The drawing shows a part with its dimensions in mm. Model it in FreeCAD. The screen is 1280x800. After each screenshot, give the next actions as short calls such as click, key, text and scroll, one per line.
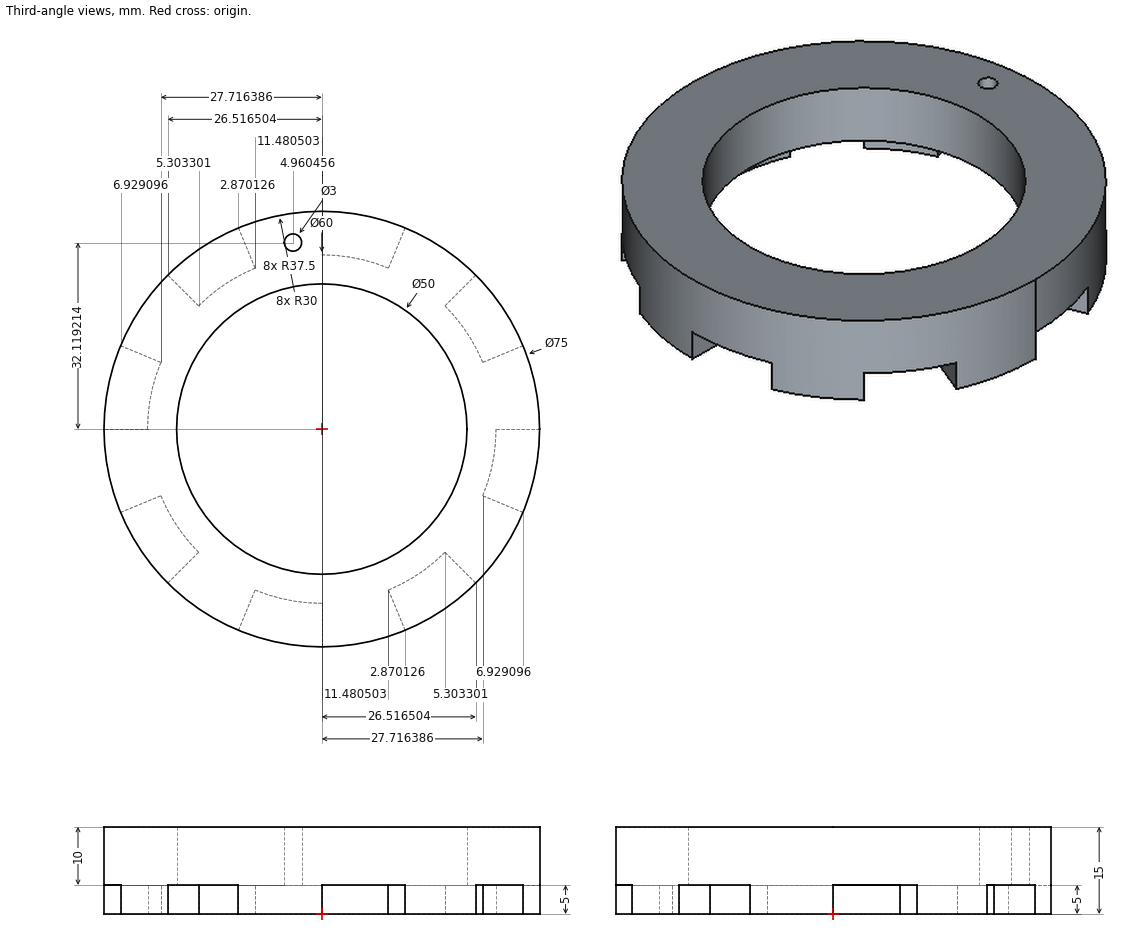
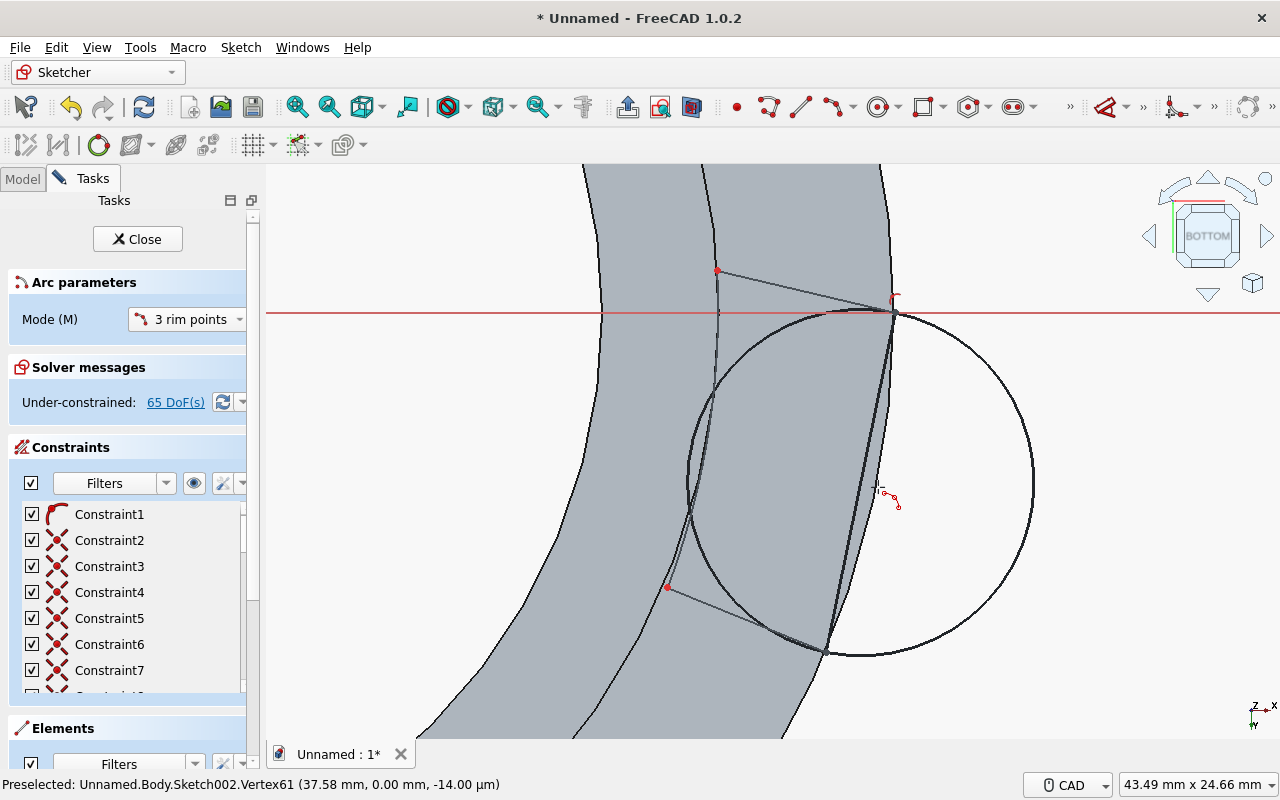
click(877, 484)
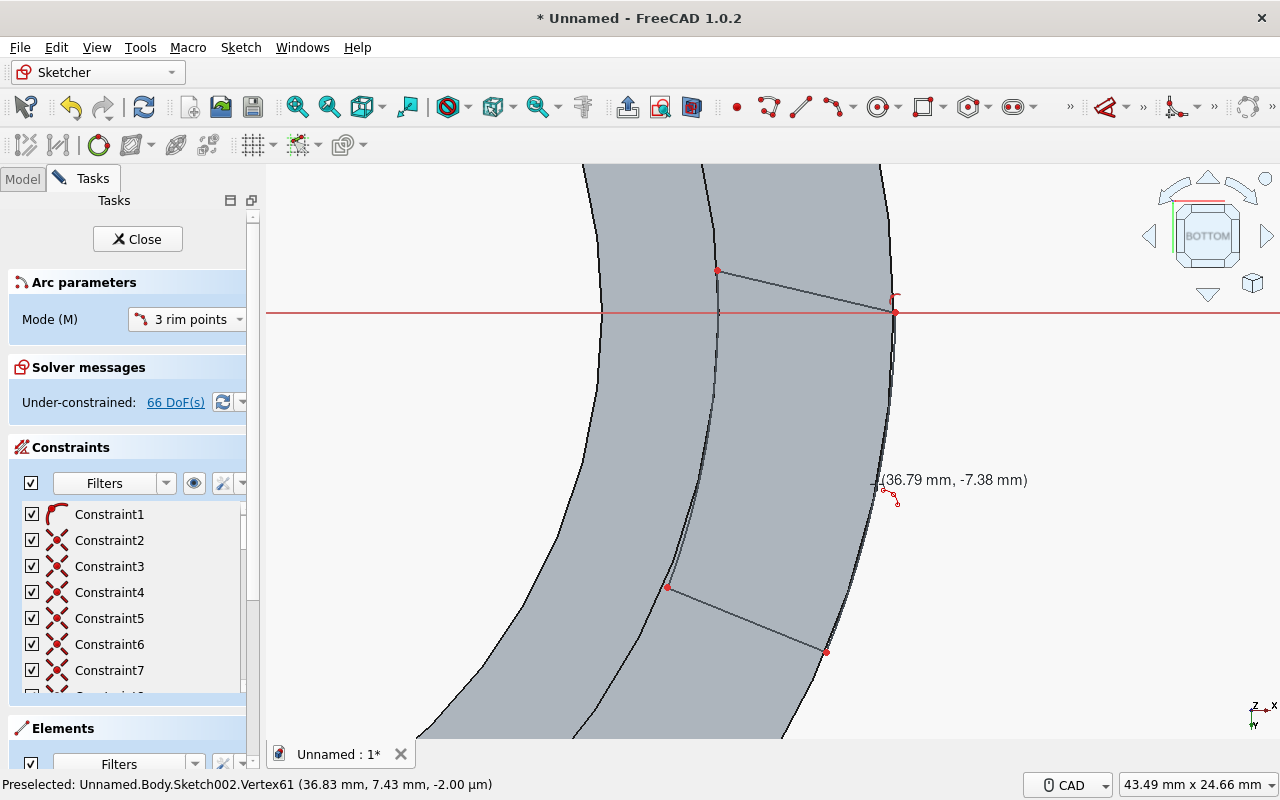
key(g)
key(l)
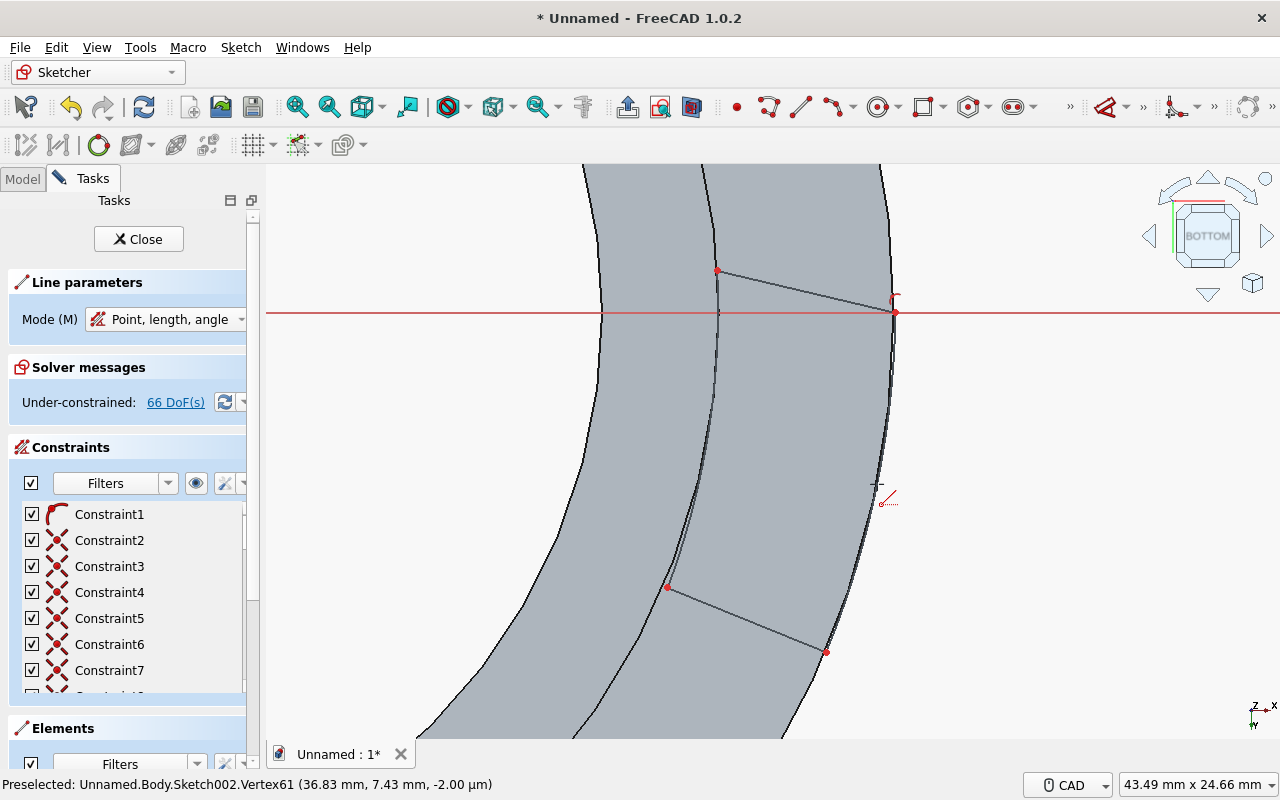
scroll(878, 487, down, 8)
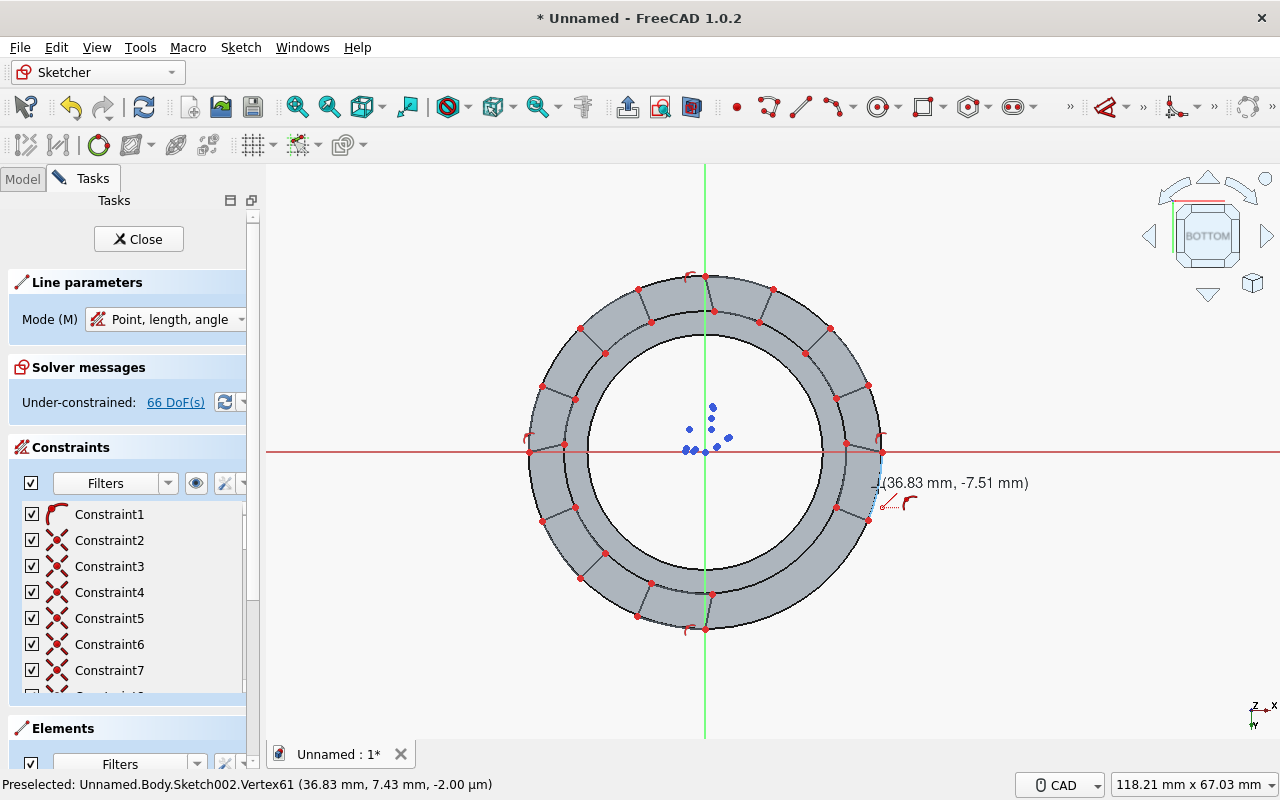
click(830, 577)
click(805, 552)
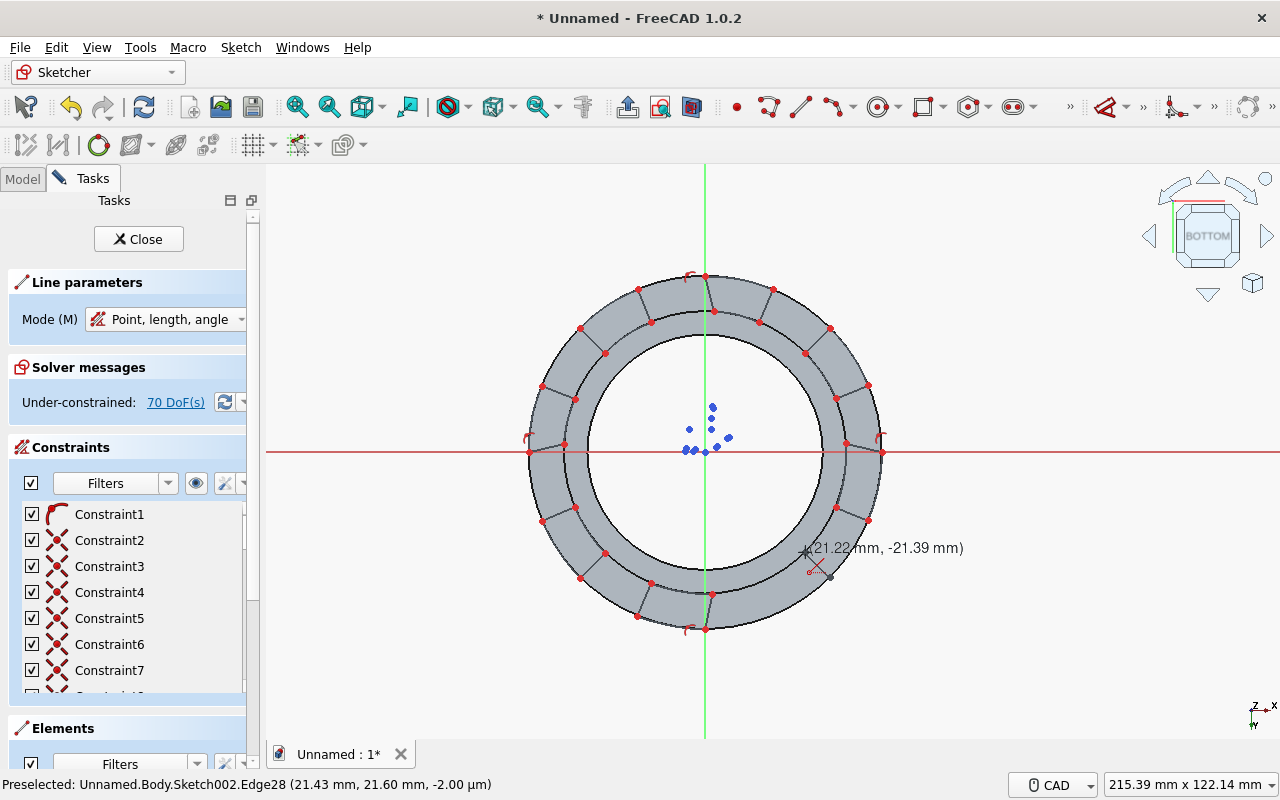
click(759, 583)
click(773, 615)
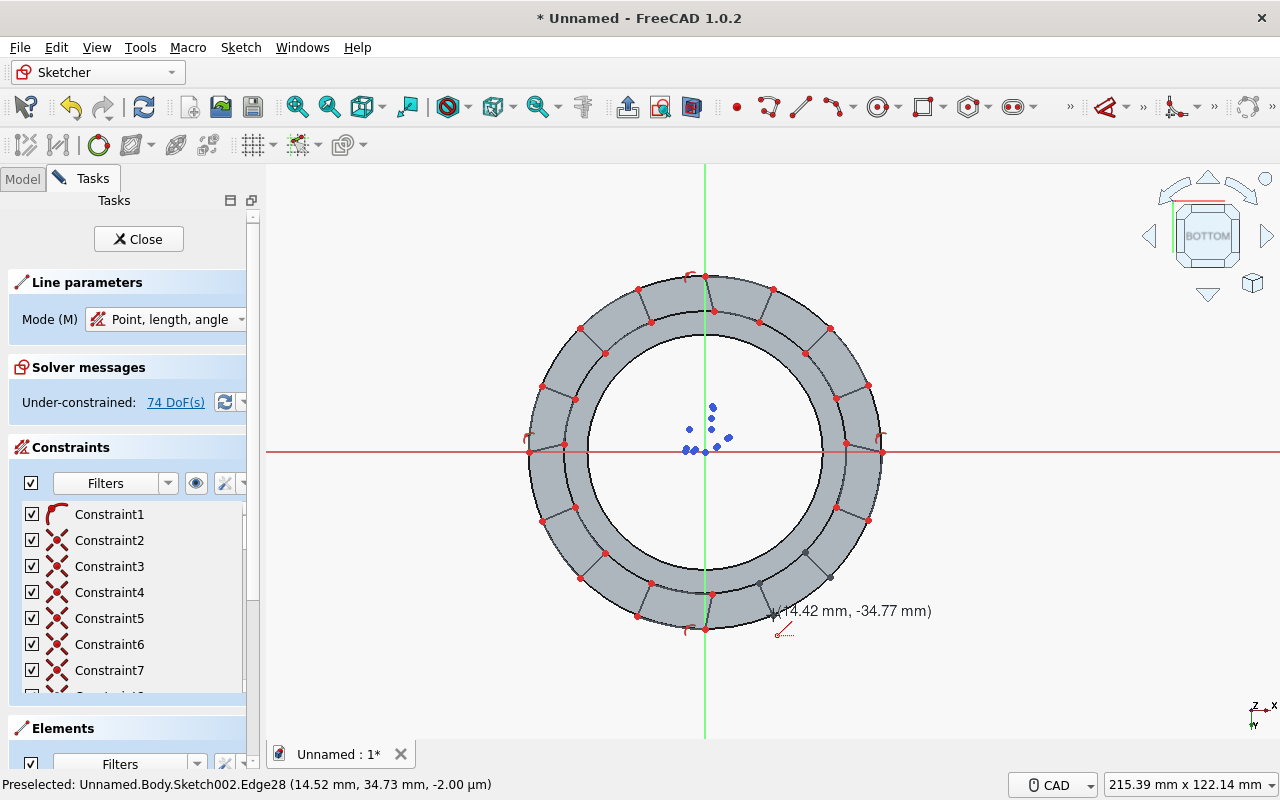
key(g)
key(3)
key(a)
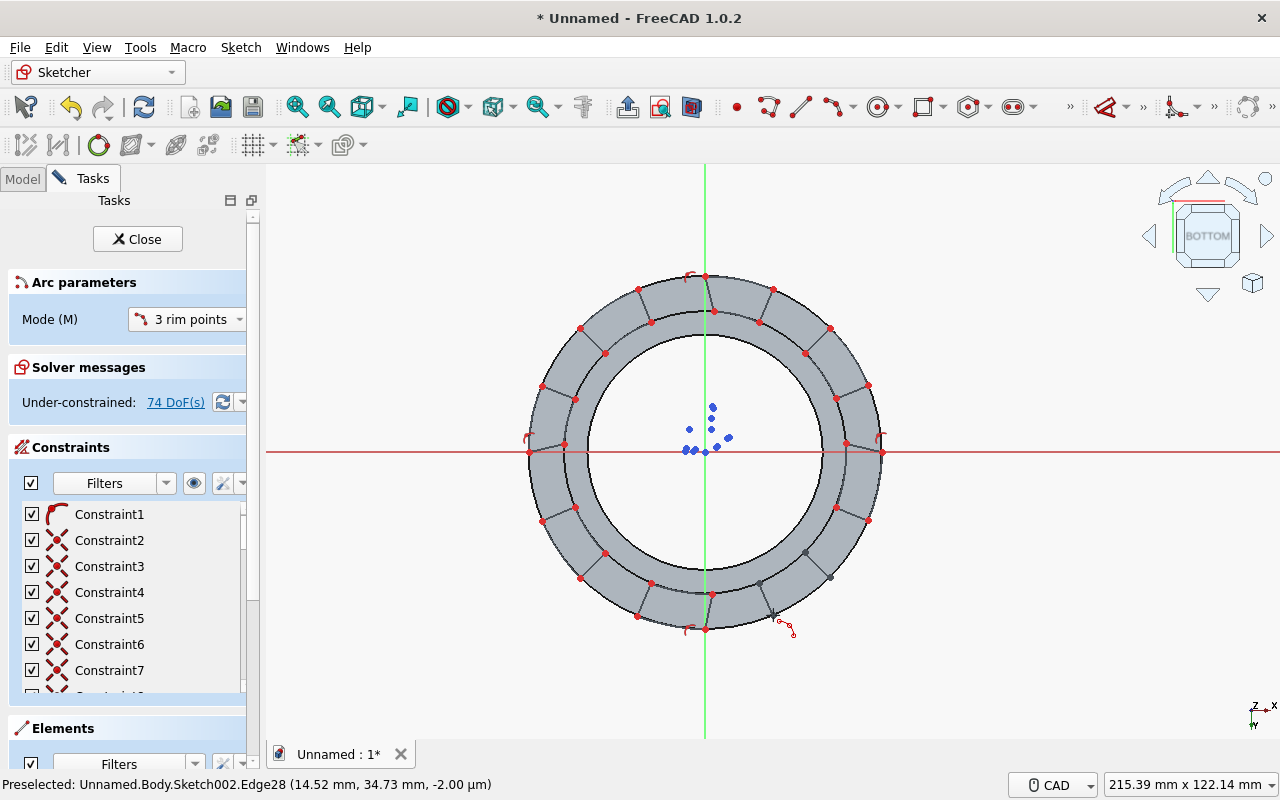
click(805, 553)
click(759, 584)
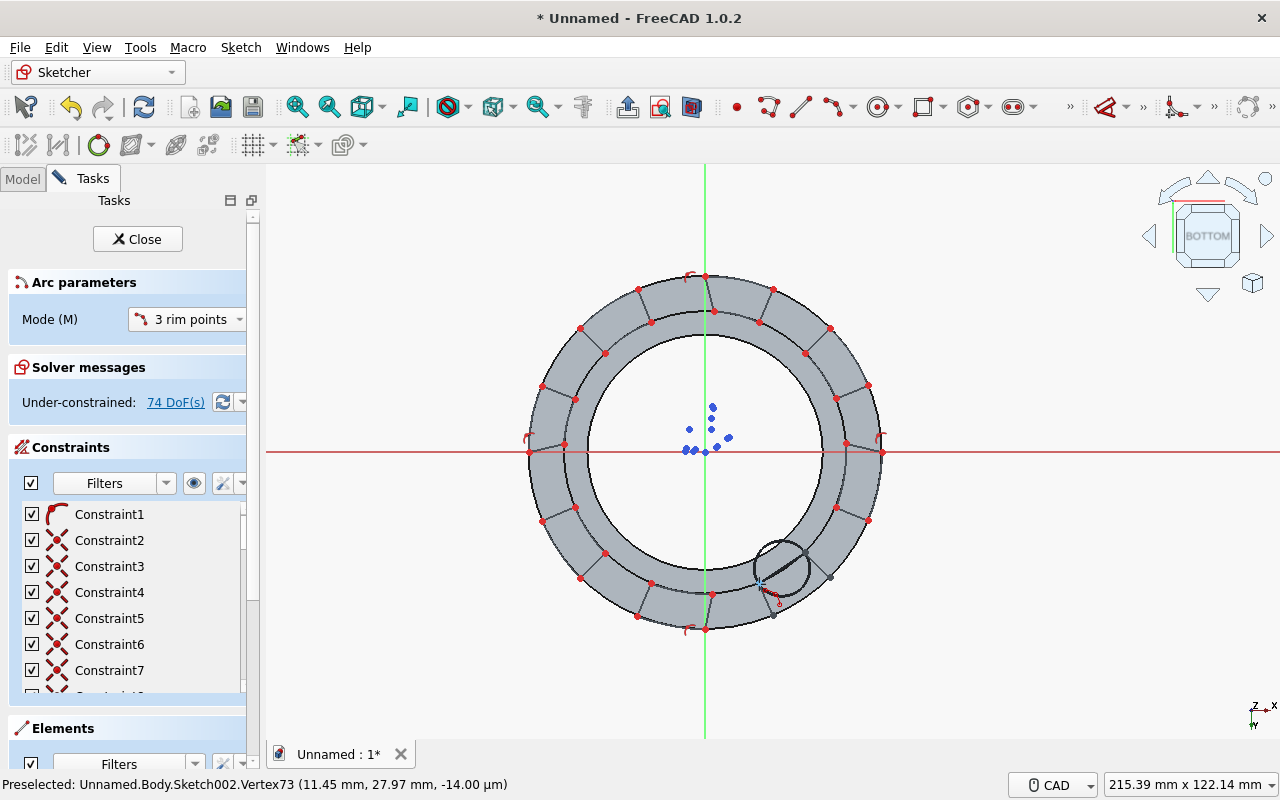
scroll(784, 570, up, 9)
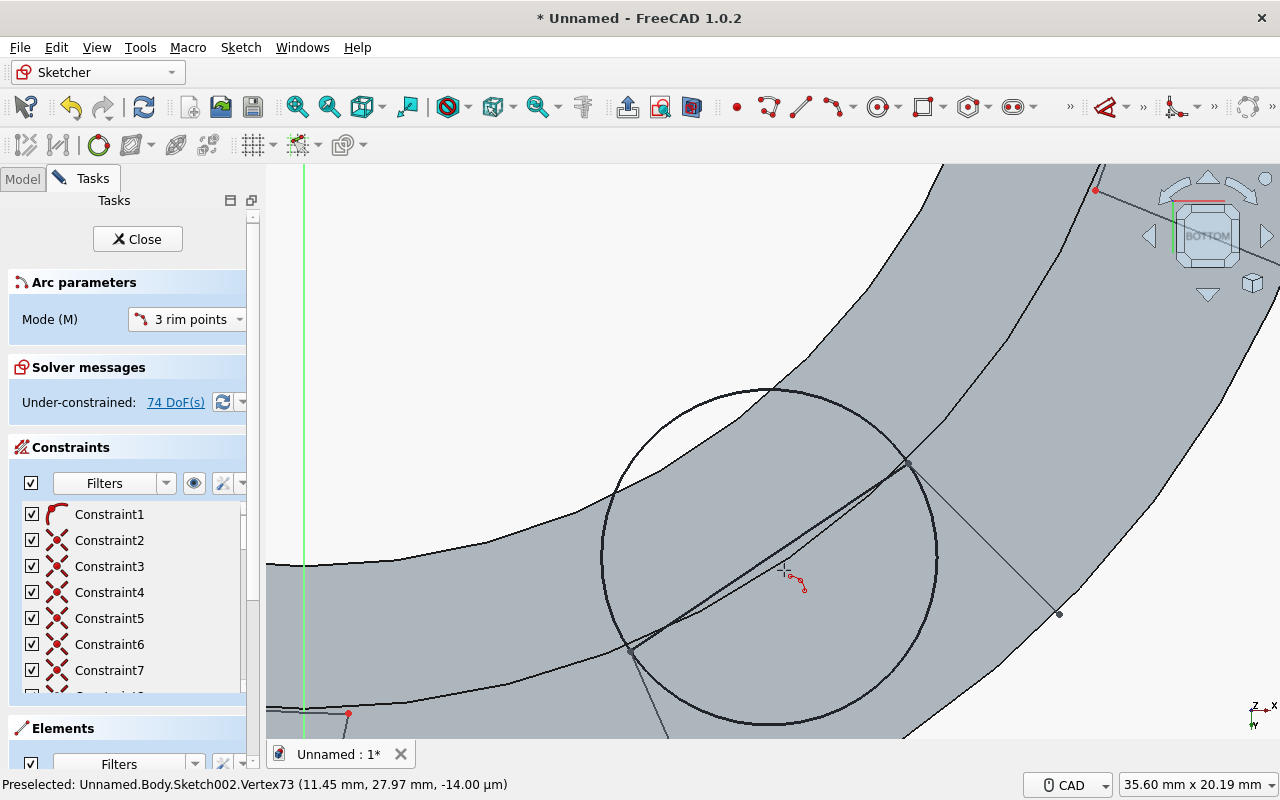
click(779, 565)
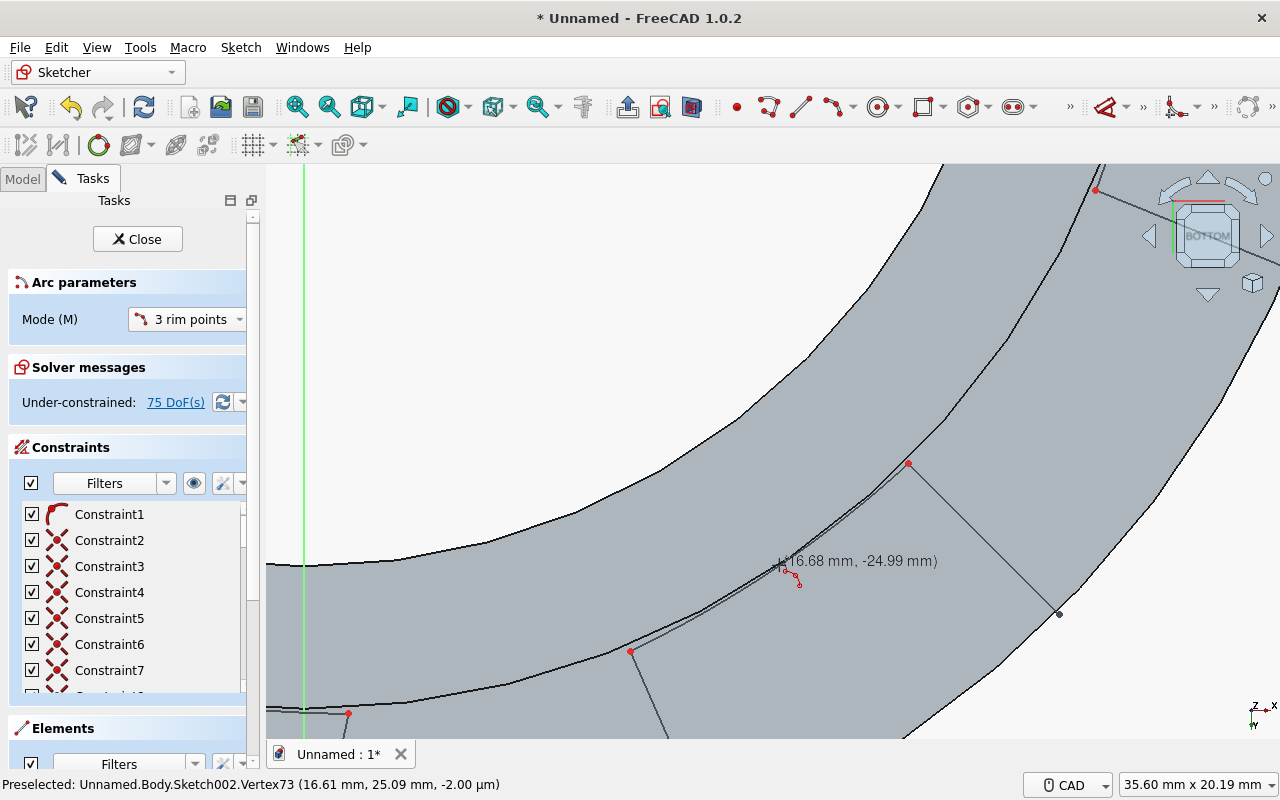
scroll(784, 570, down, 9)